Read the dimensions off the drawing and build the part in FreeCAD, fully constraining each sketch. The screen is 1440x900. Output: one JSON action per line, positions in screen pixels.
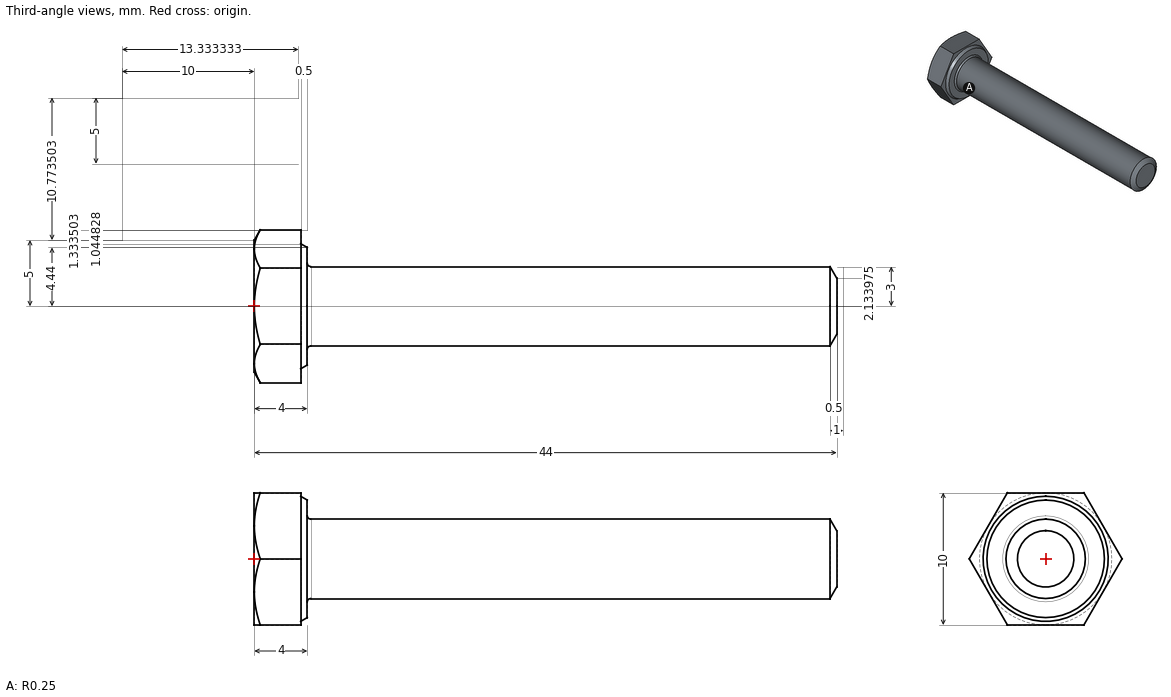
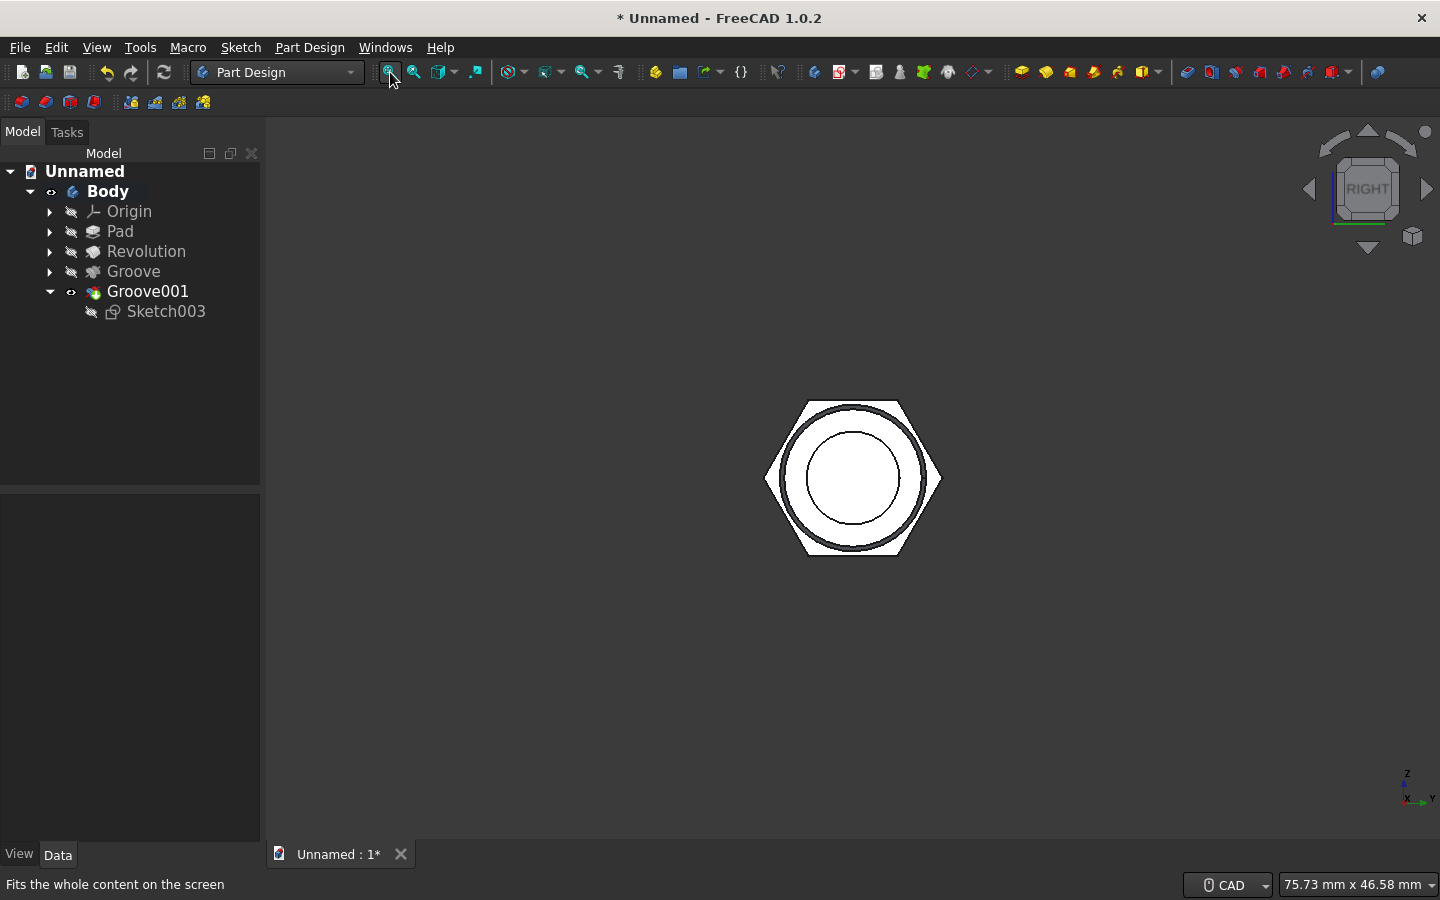
{"action": "key", "text": "5"}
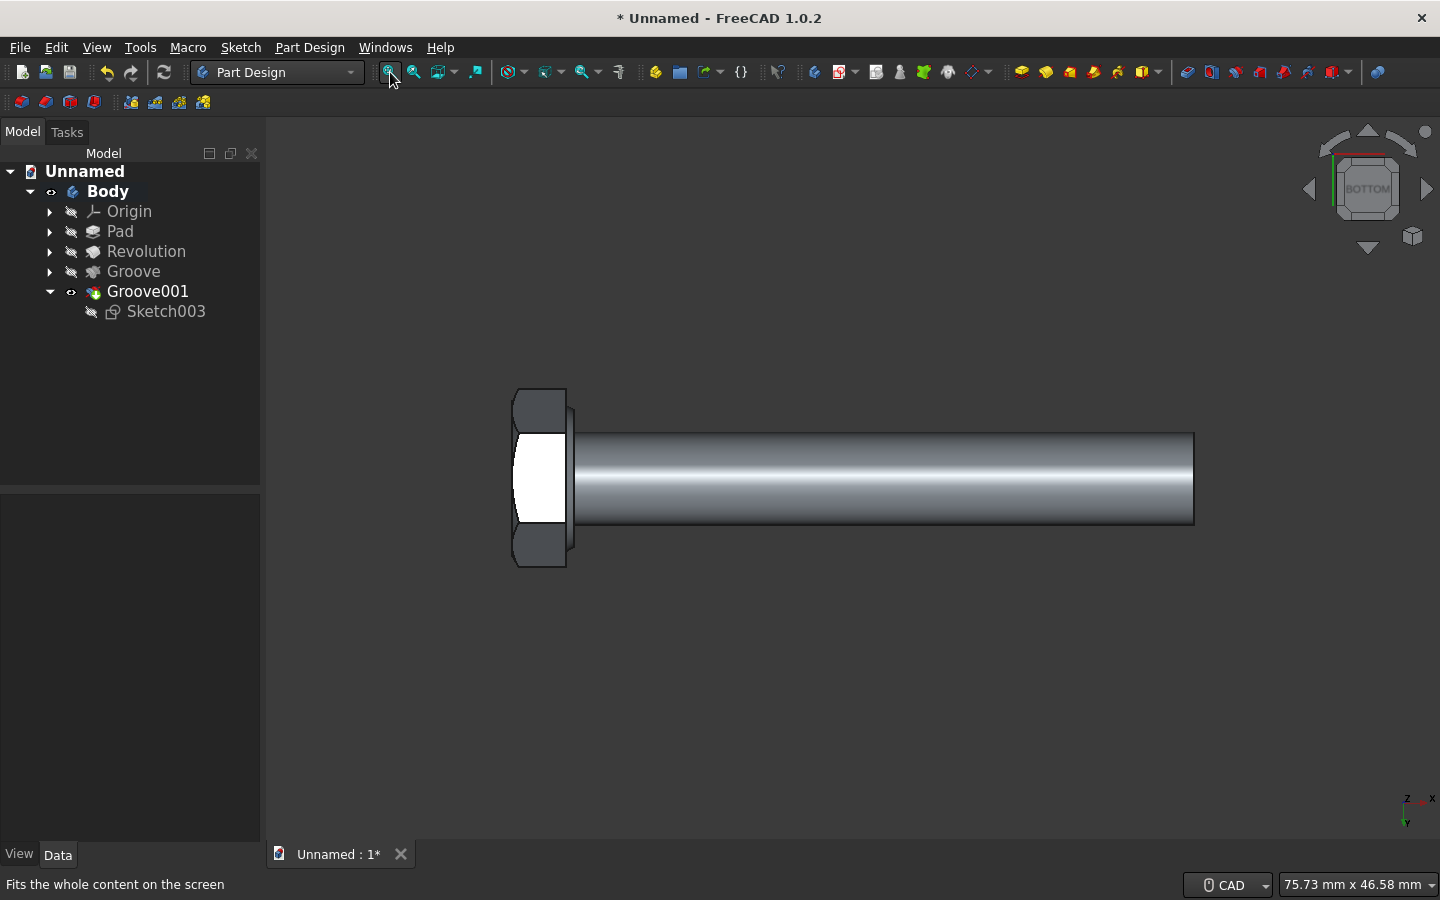
{"action": "key", "text": "4"}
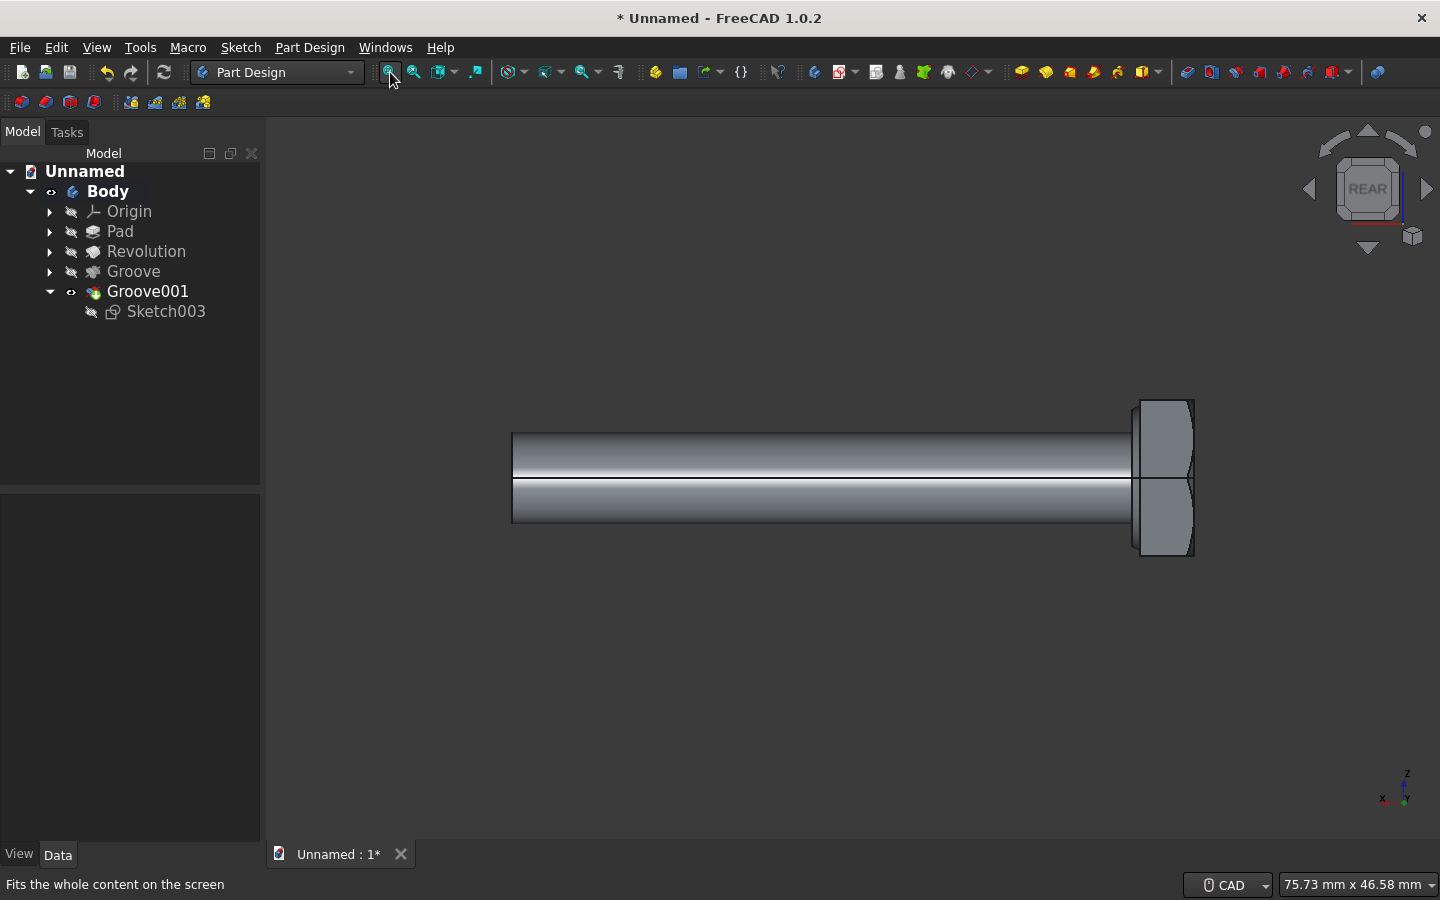
{"action": "key", "text": "6"}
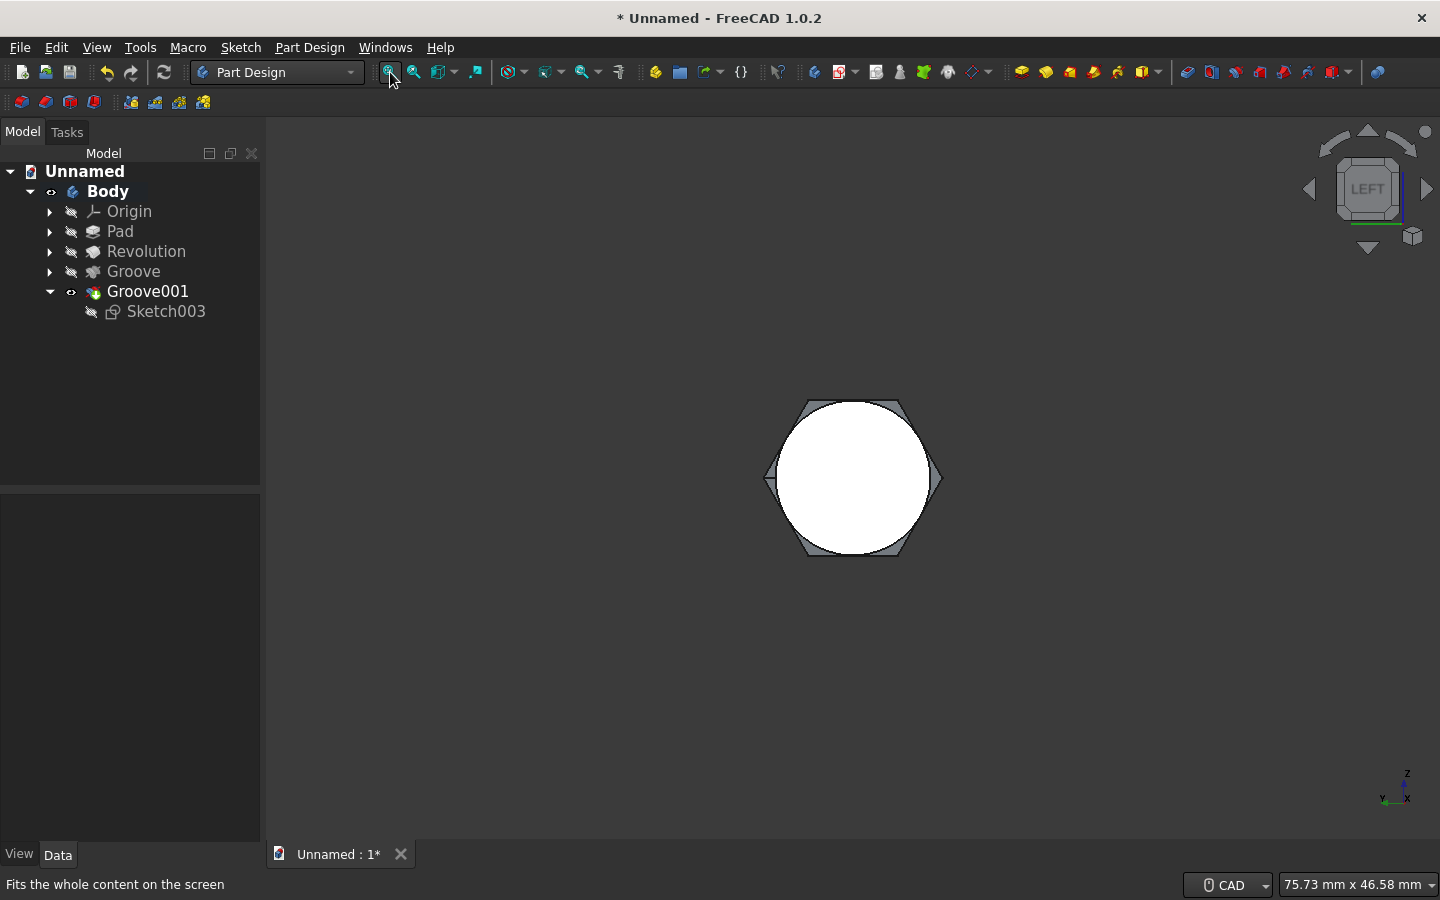
{"action": "left_click", "coordinate": [390, 72]}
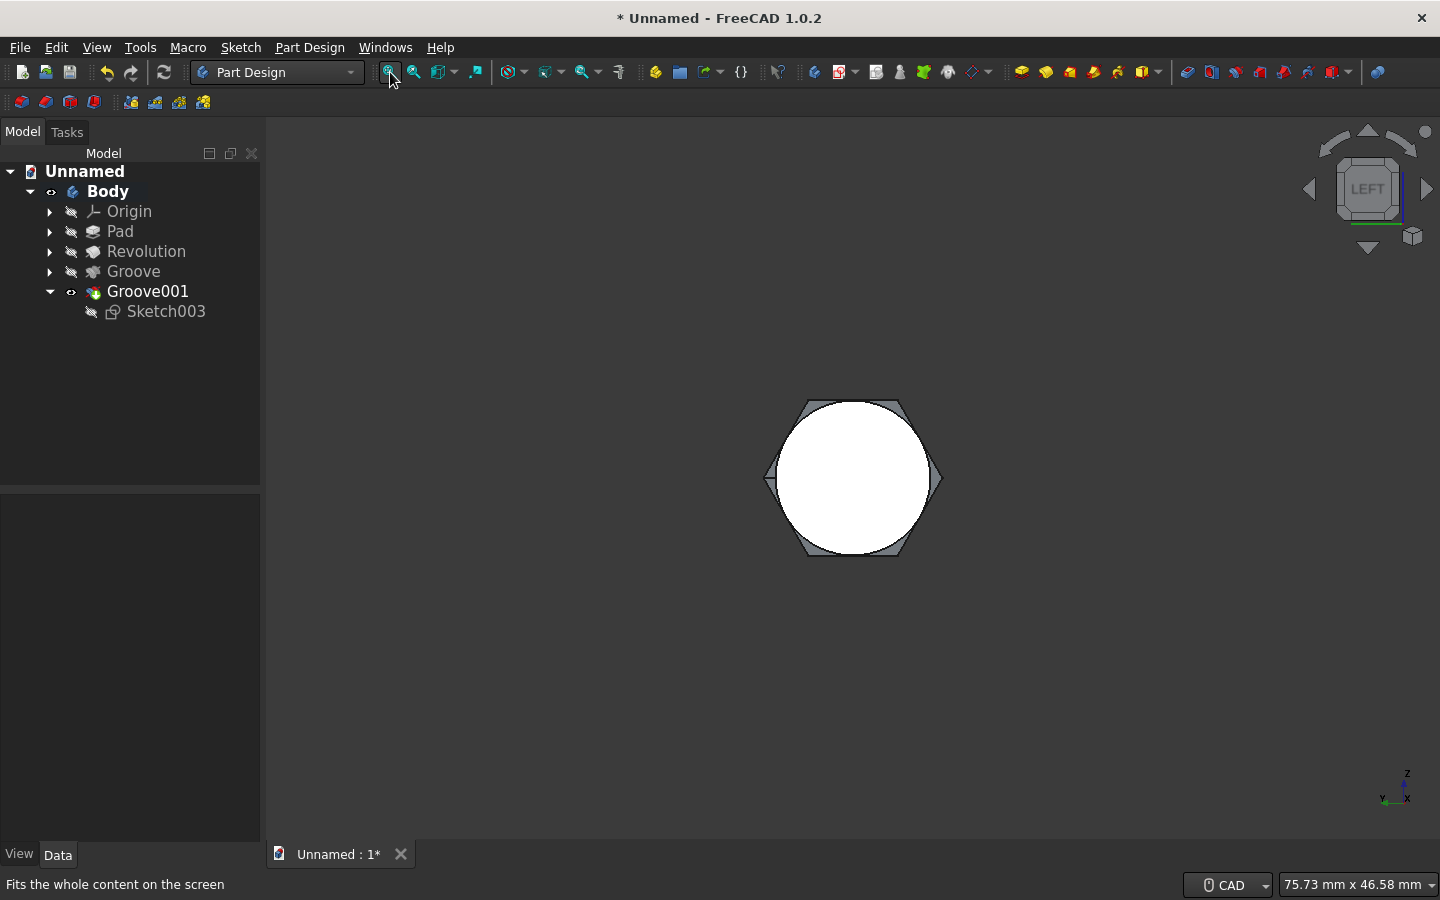
{"action": "key", "text": "v 3"}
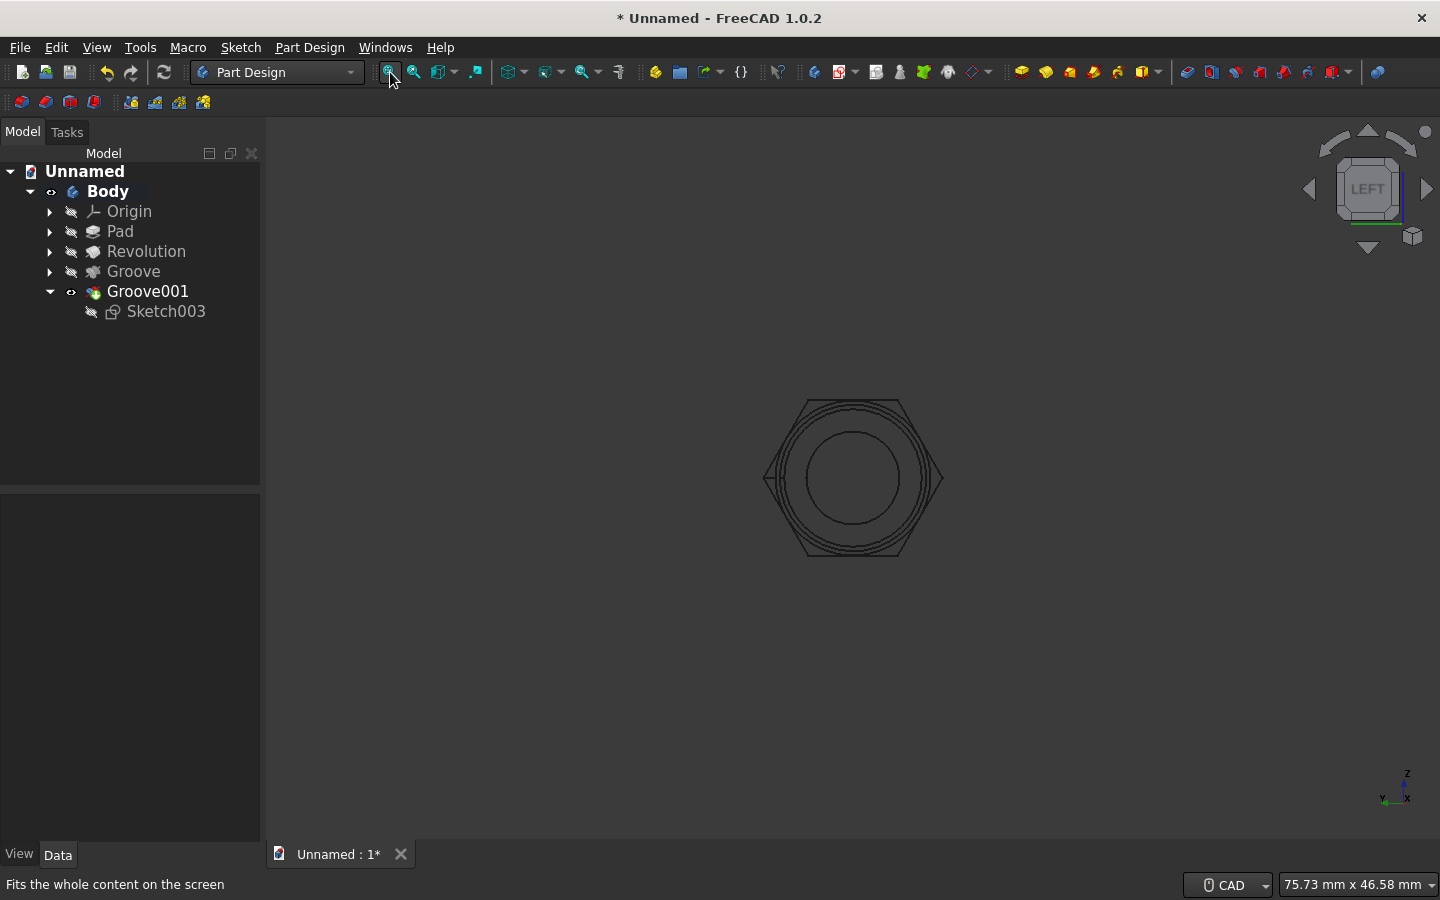
{"action": "key", "text": "0"}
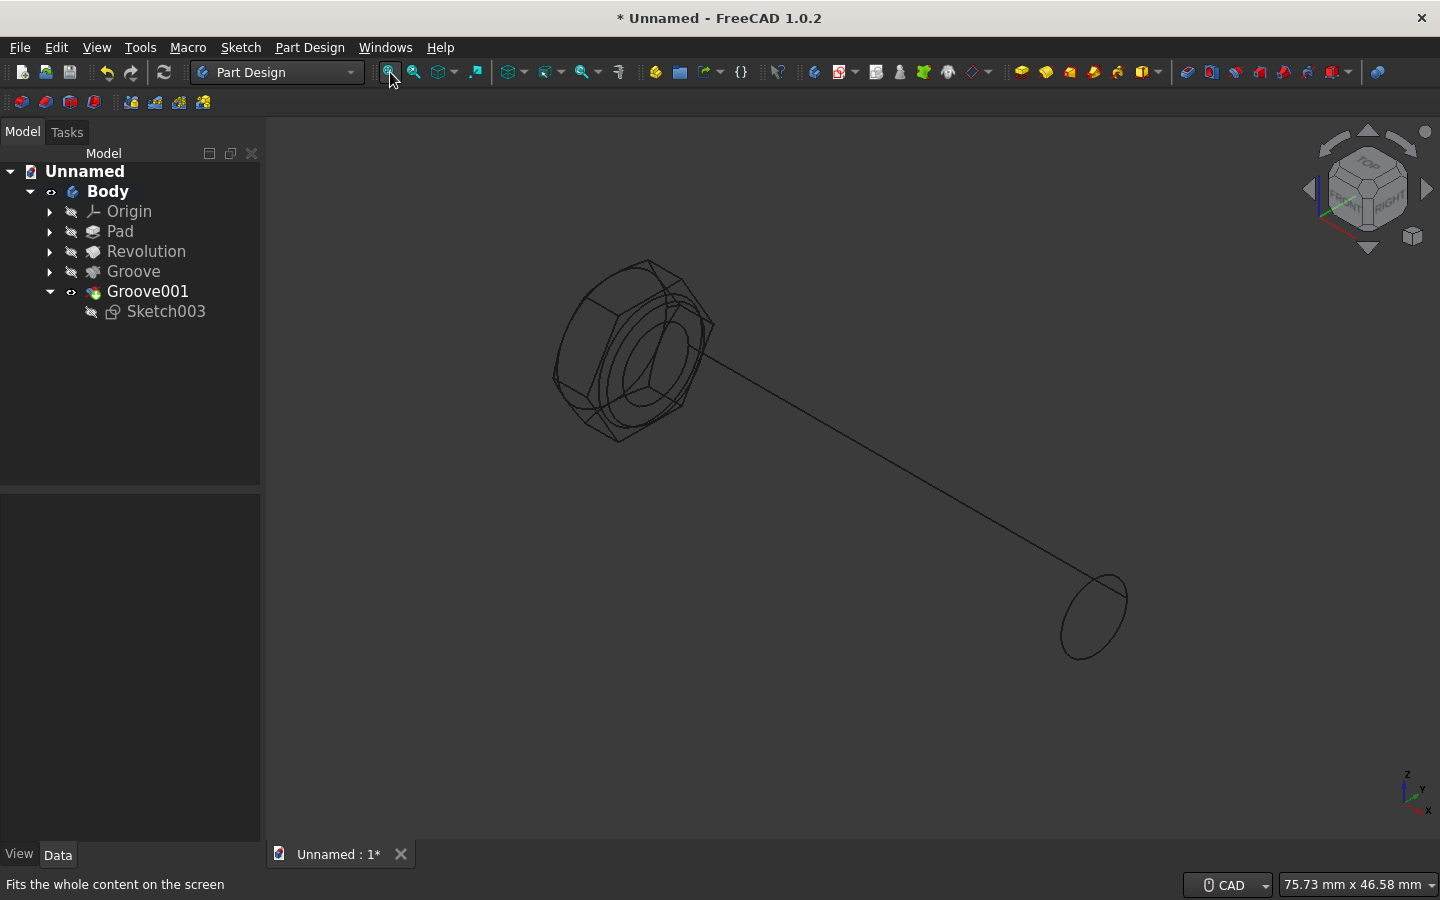
{"action": "left_click", "coordinate": [623, 382]}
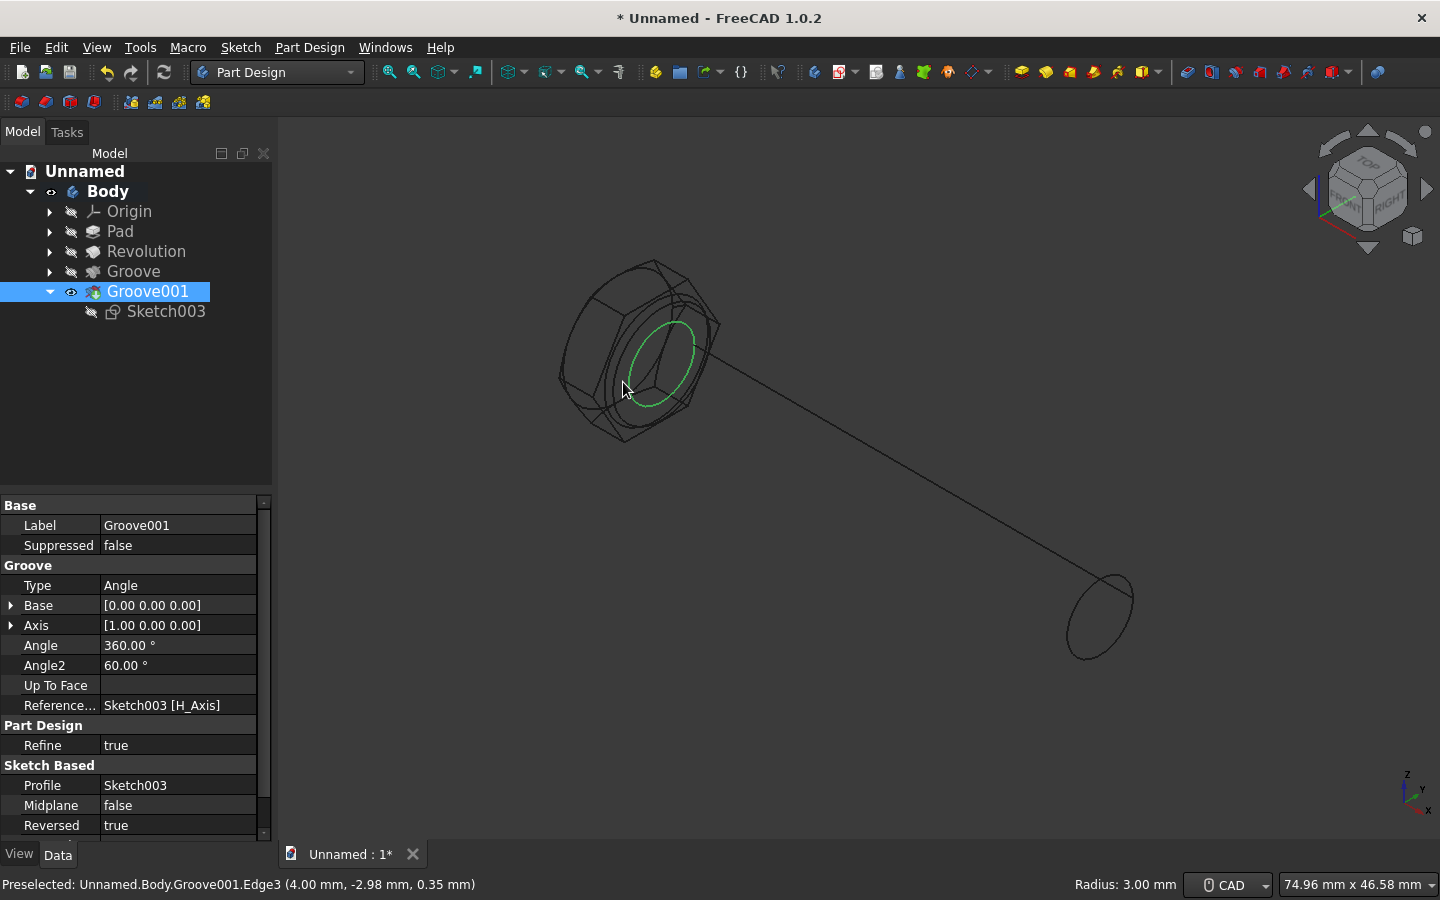
{"action": "key", "text": "v 1"}